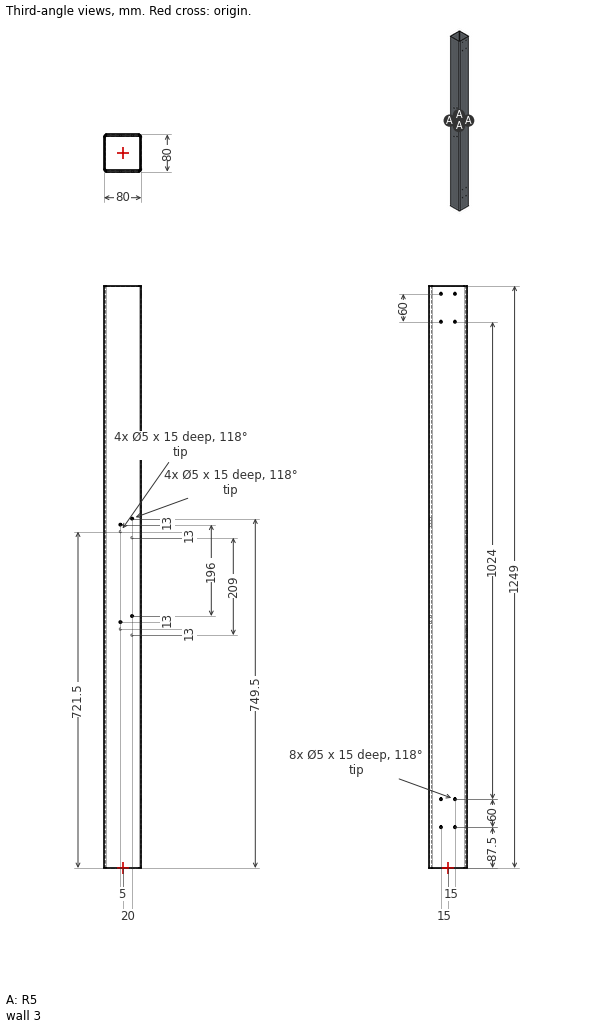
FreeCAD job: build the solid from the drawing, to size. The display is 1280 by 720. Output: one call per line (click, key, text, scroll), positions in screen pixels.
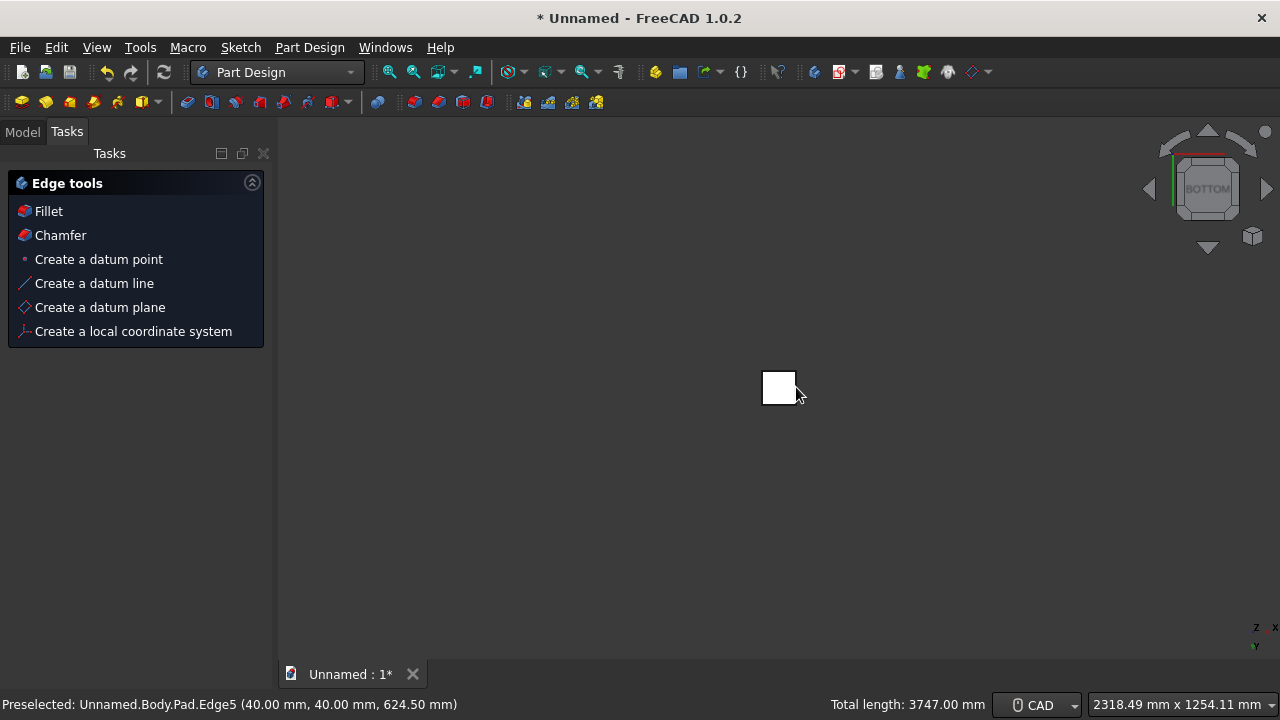
key(4)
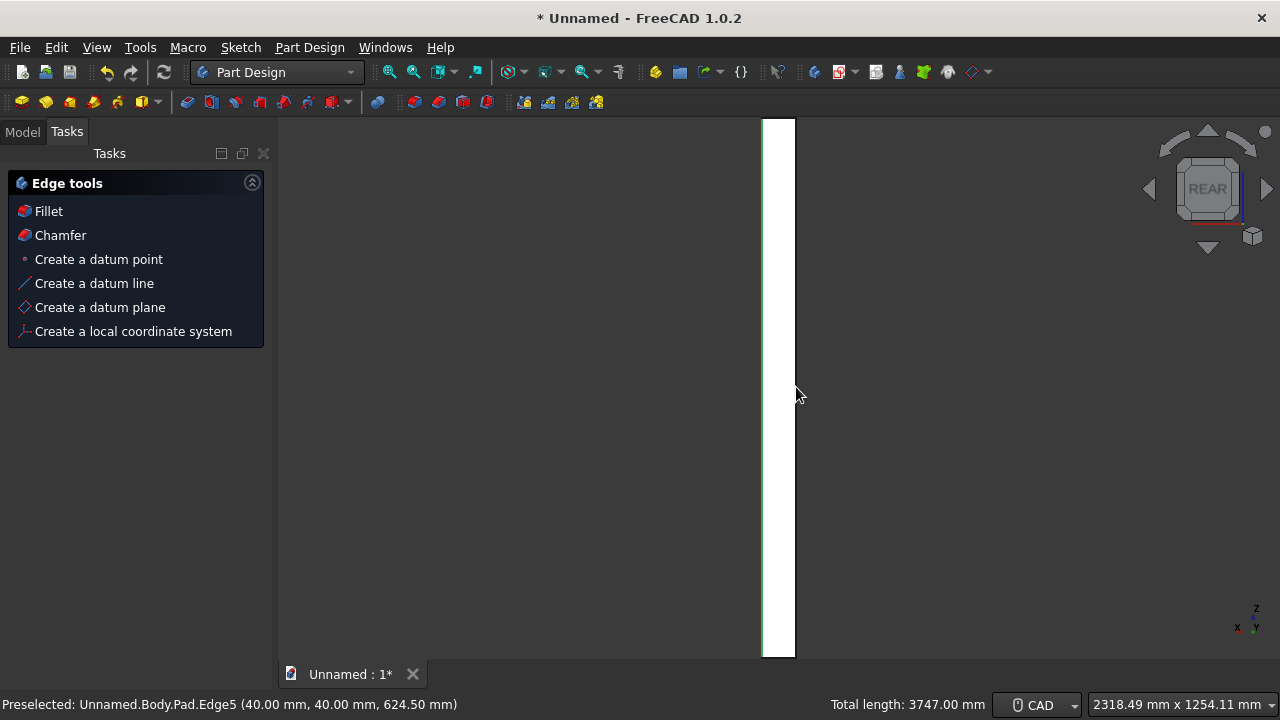
click(796, 387, ctrl)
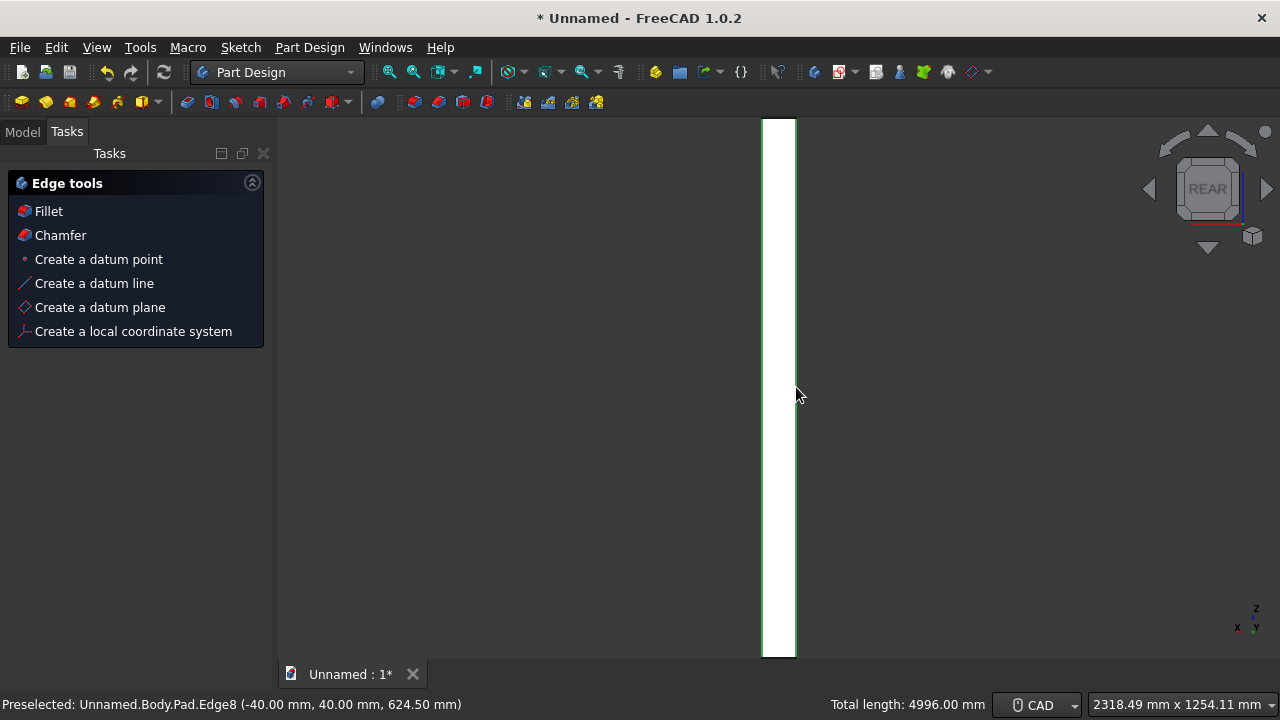
click(416, 102)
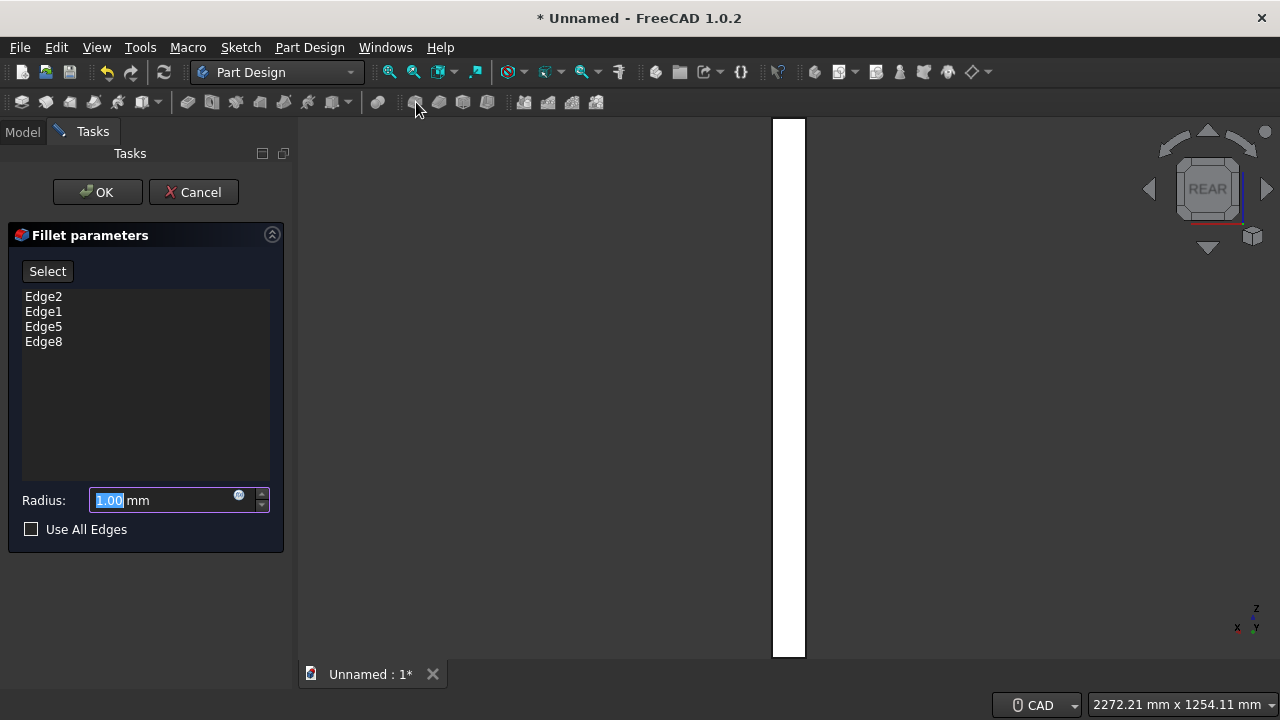
text(5)
key(Tab)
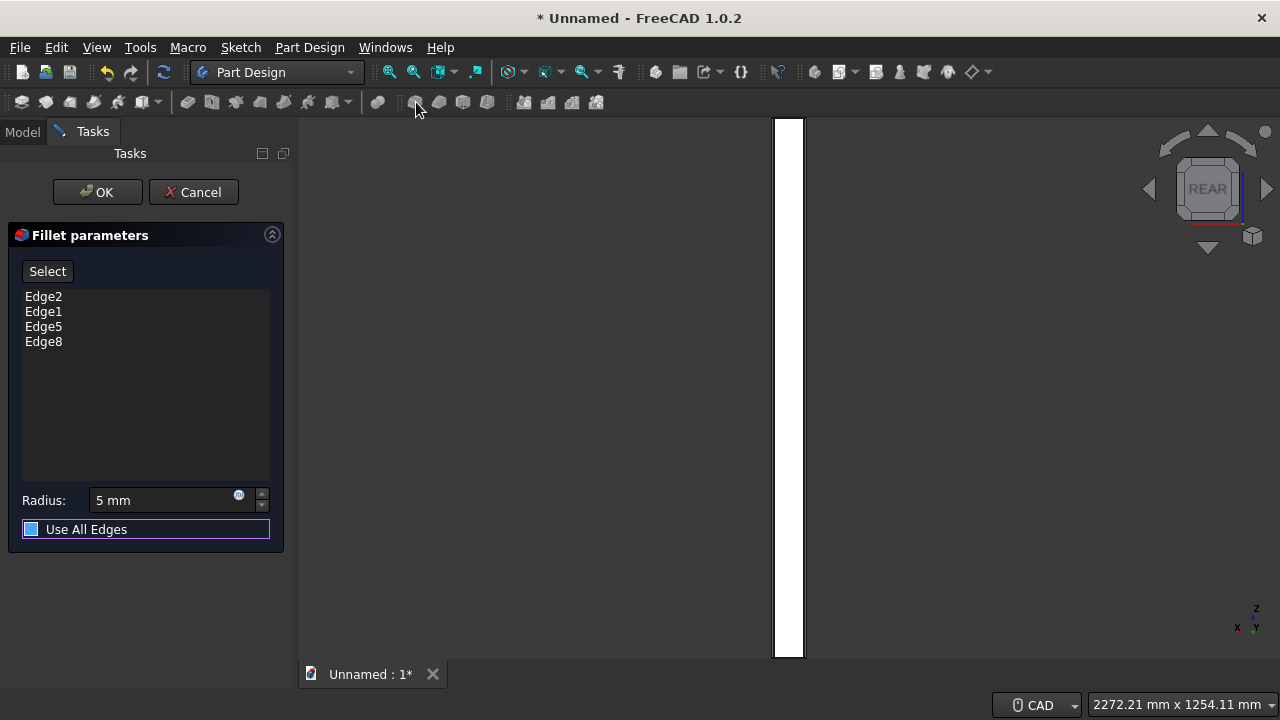
click(98, 192)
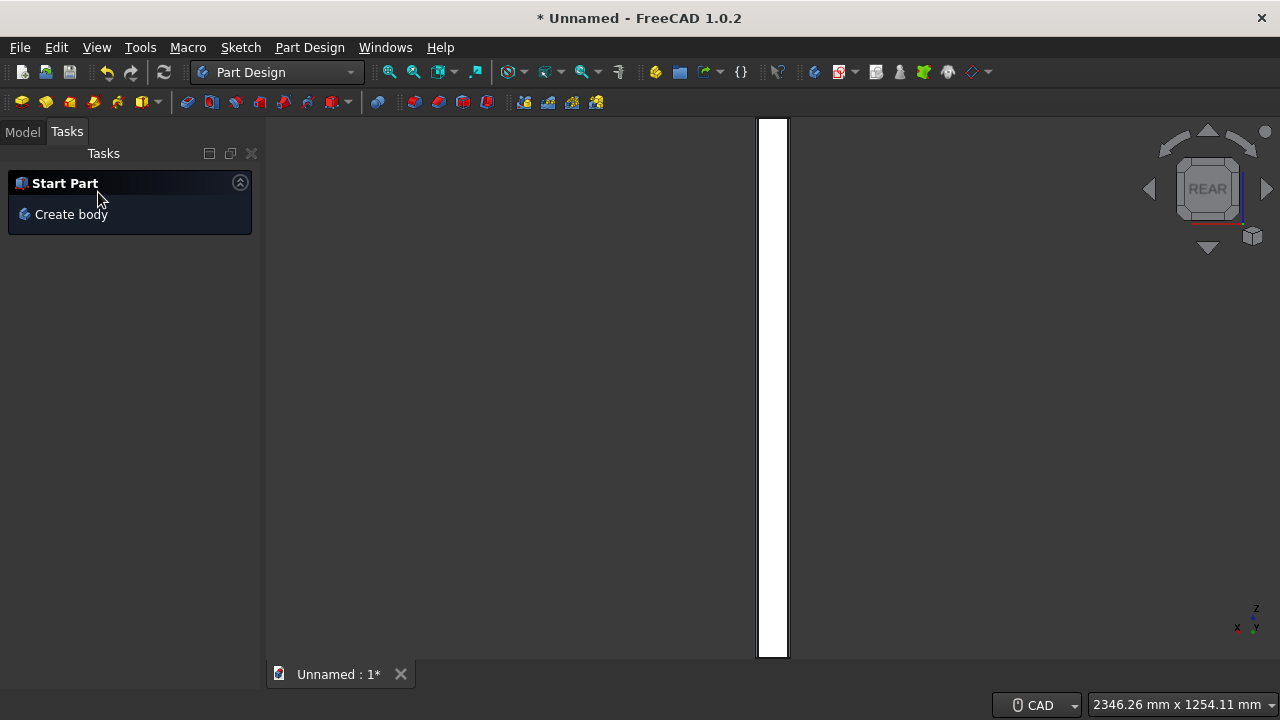
key(0)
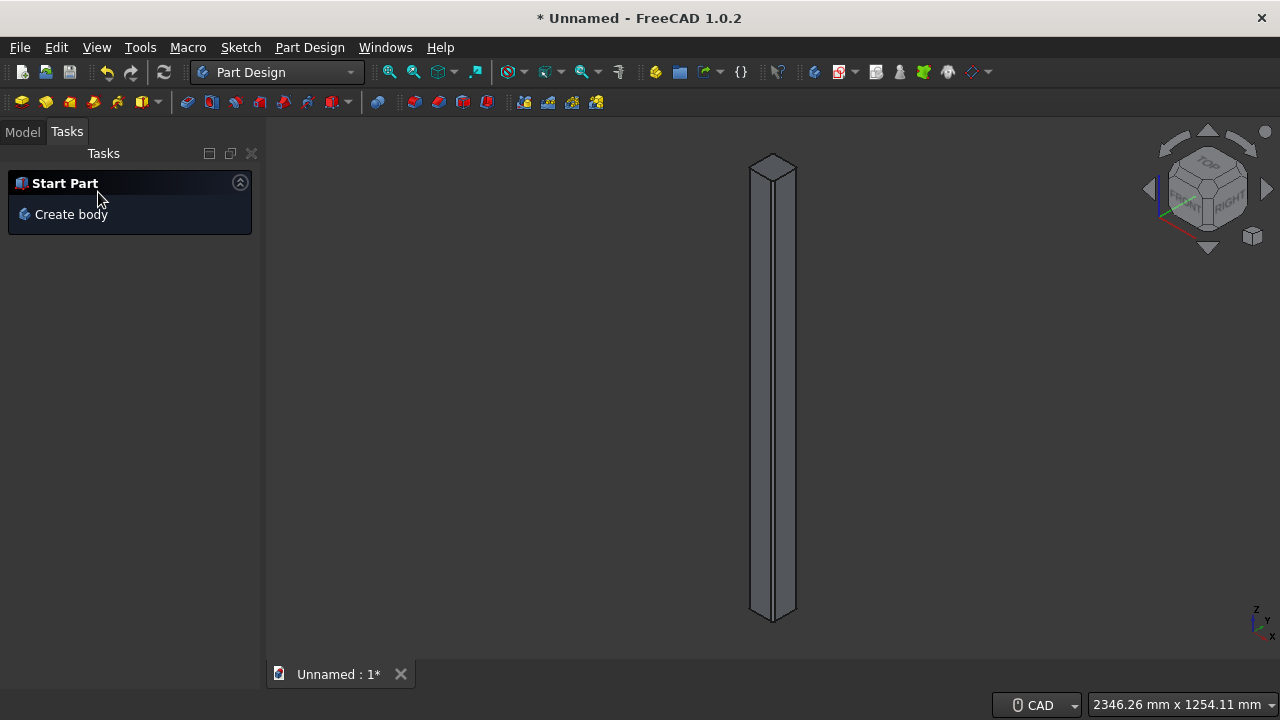
click(773, 167)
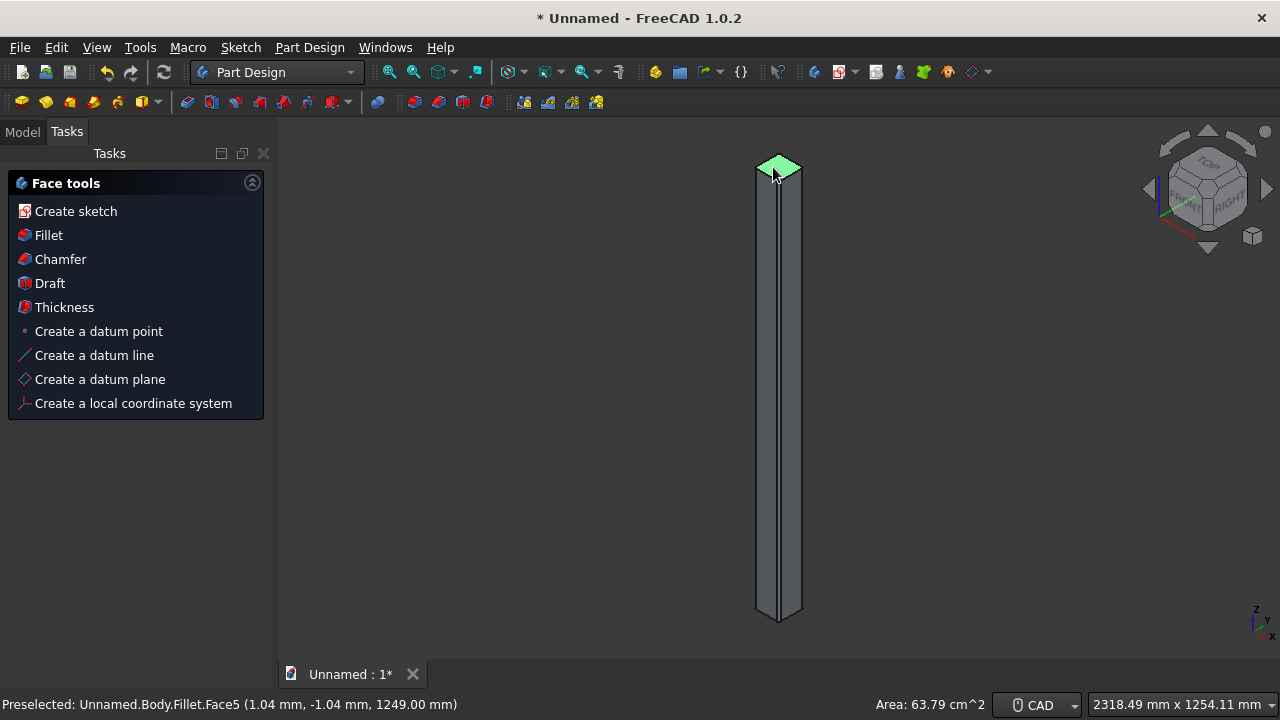
key(2)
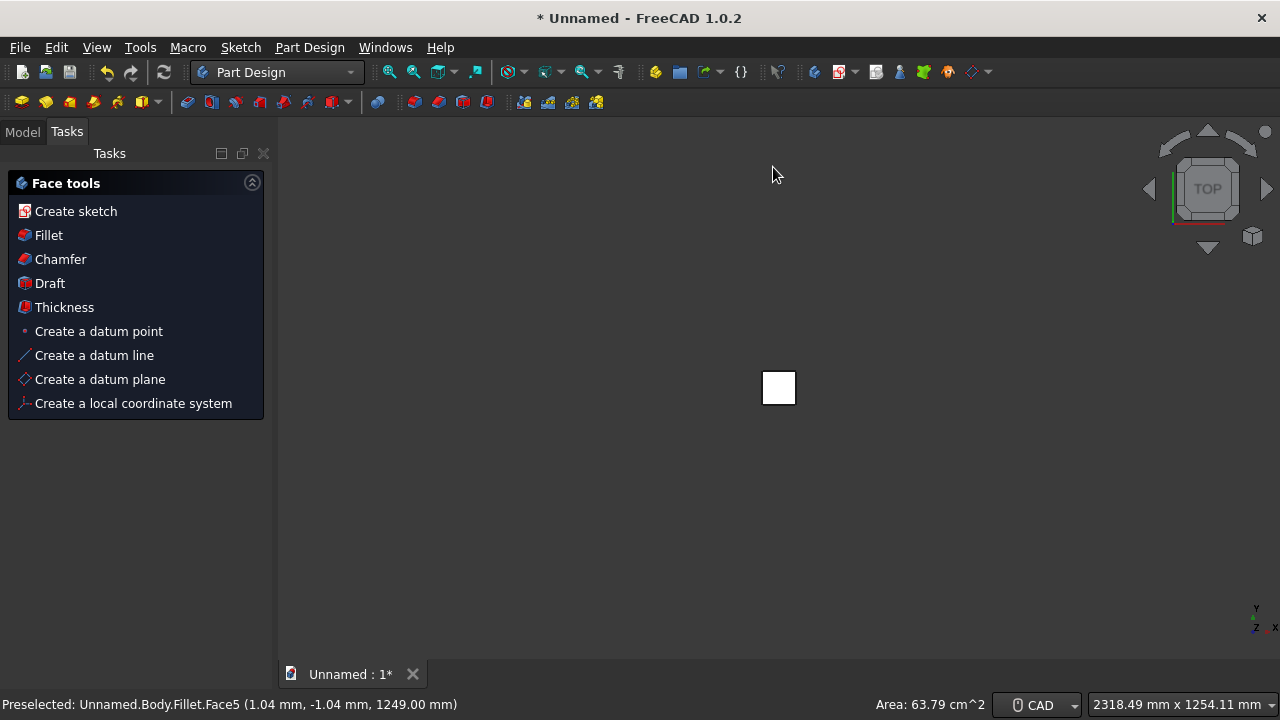
key(v)
key(f)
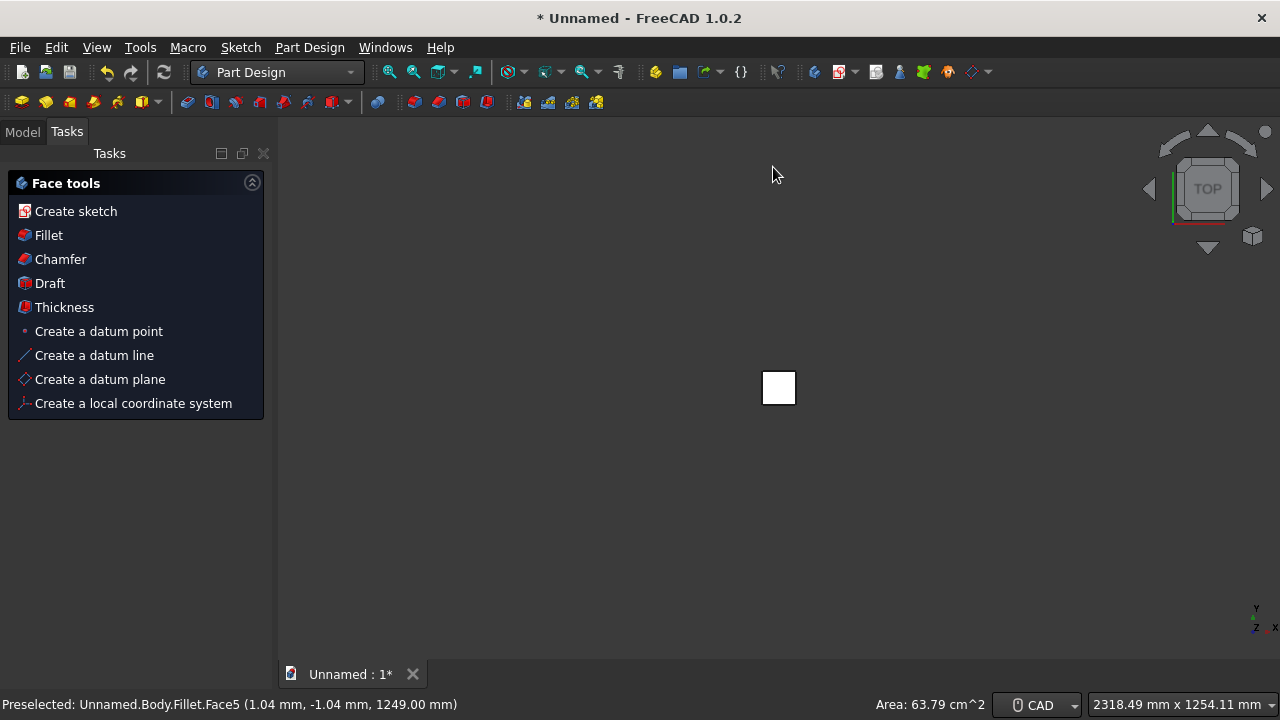
key(1)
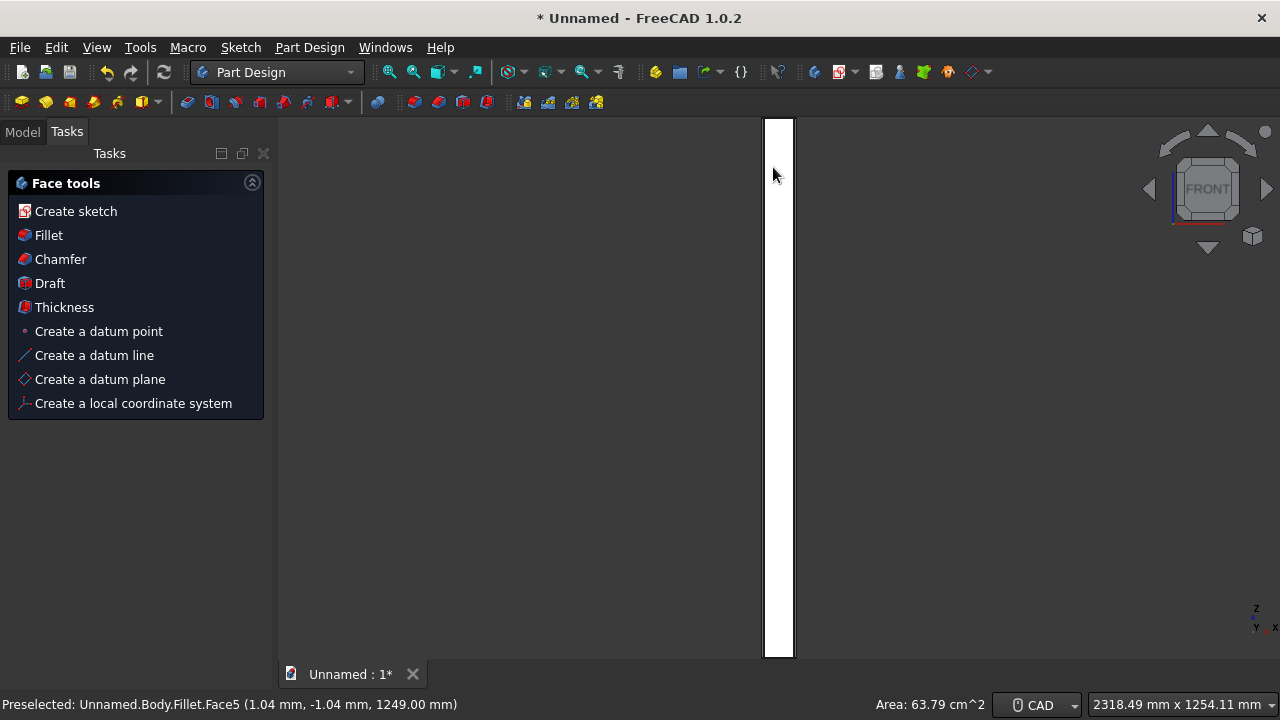
key(3)